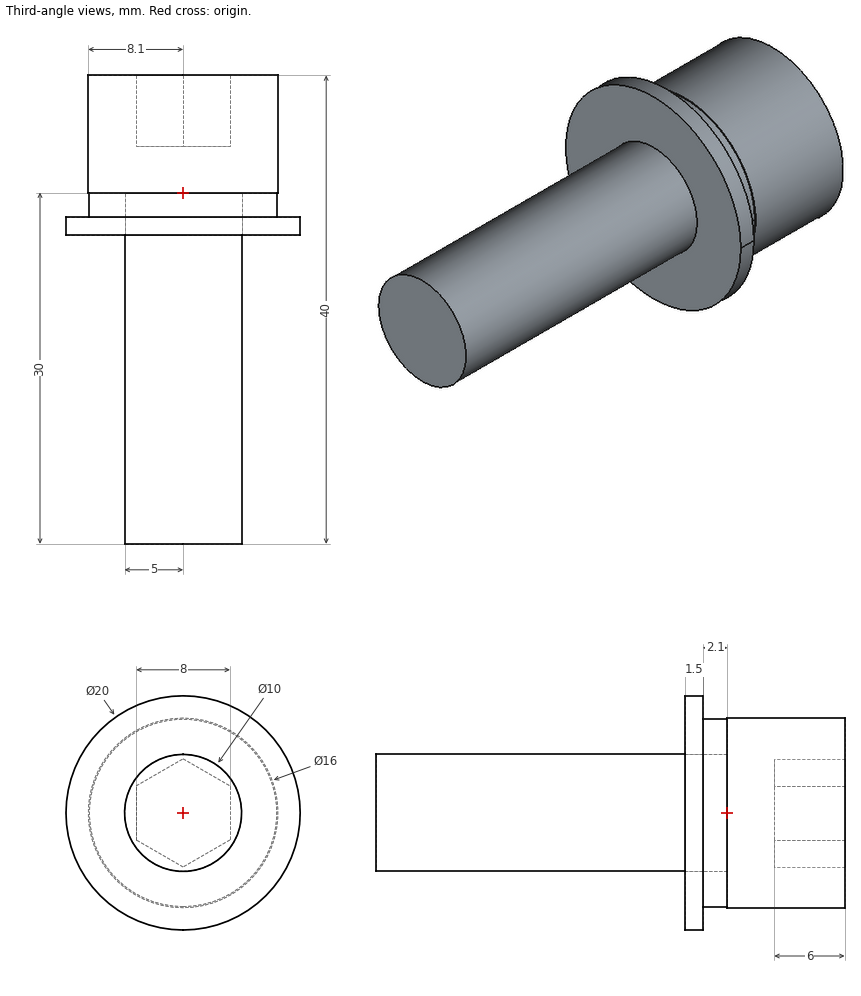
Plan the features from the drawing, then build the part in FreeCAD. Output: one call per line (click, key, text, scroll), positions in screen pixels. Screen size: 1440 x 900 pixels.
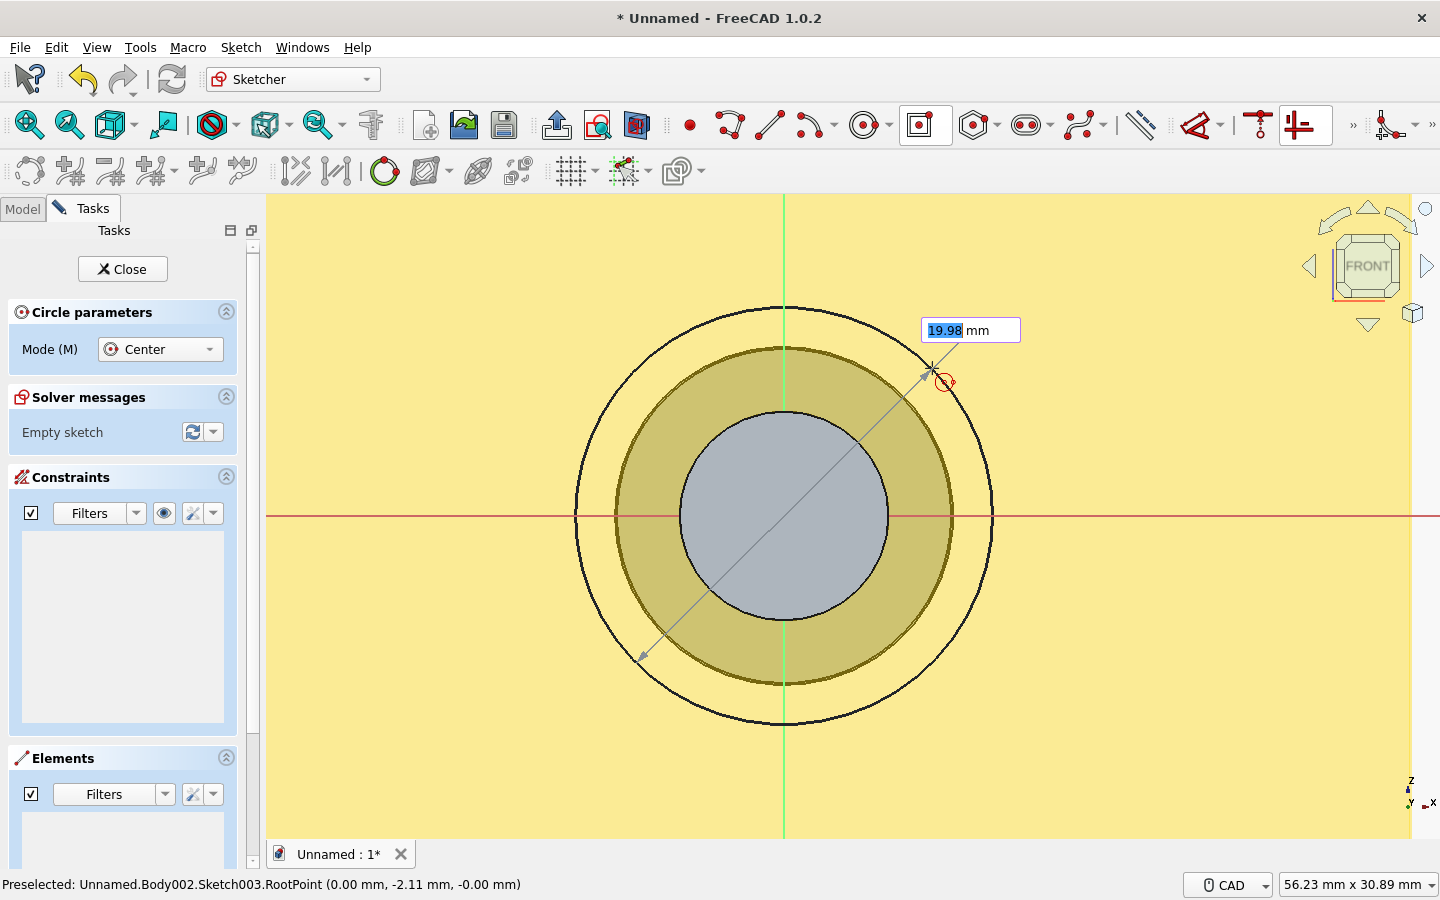
text(20)
key(Return)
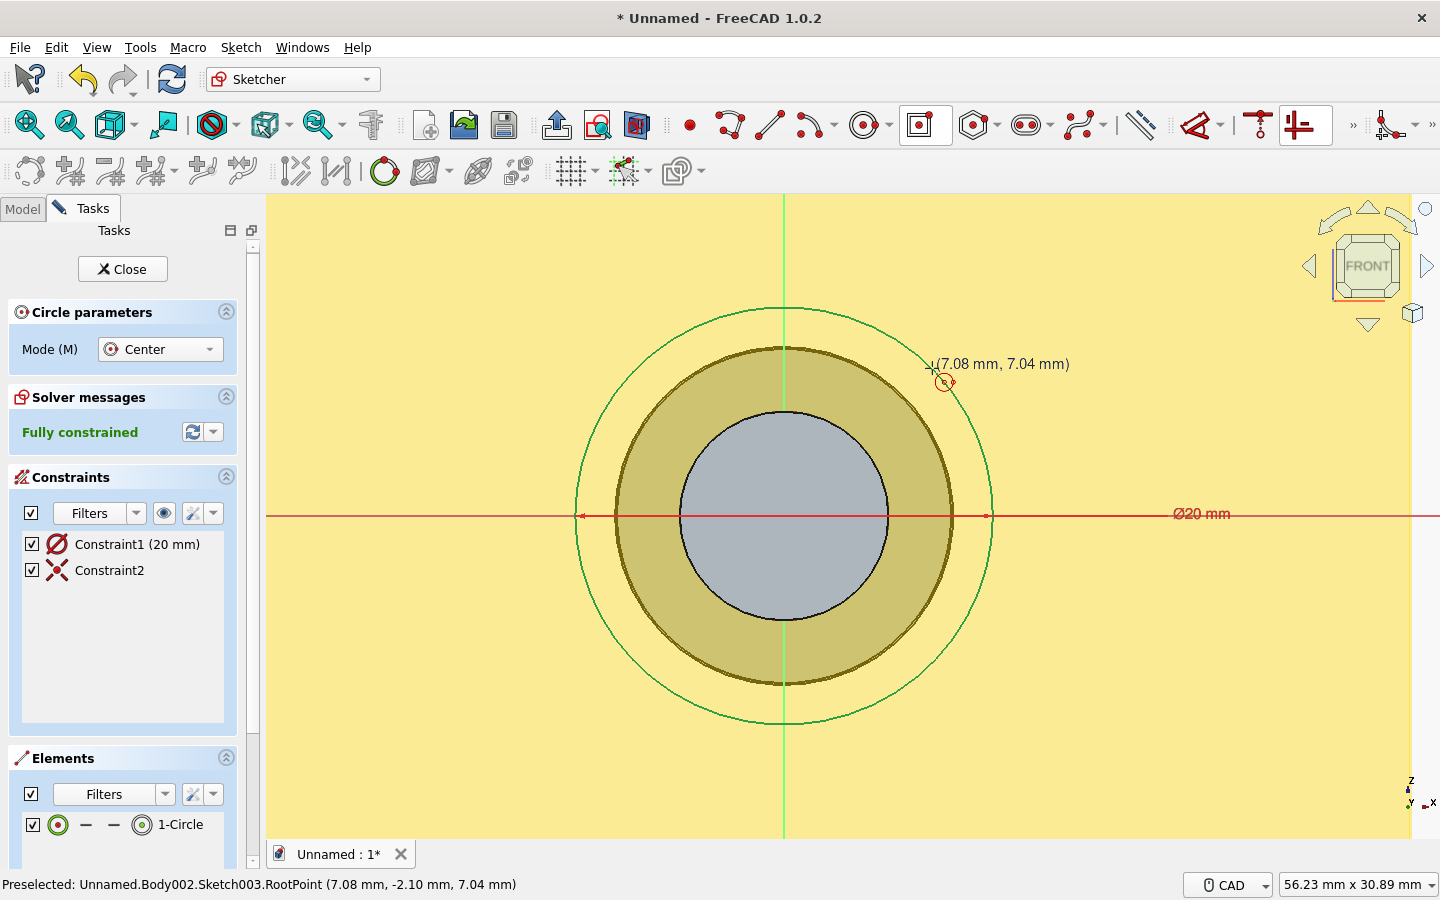
click(784, 516)
move(858, 442)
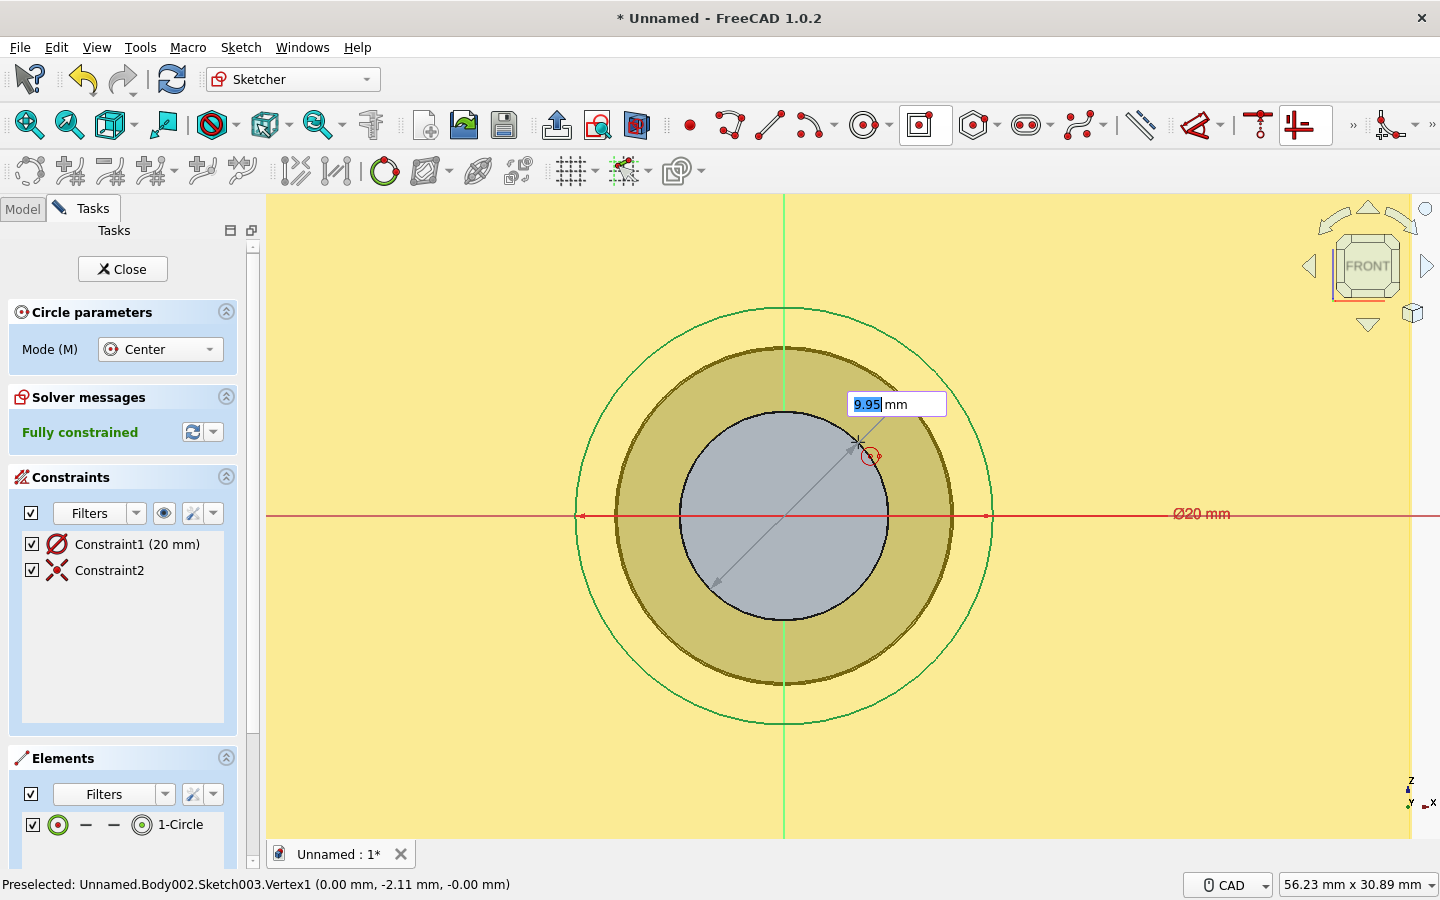
text(10)
key(Return)
key(Escape)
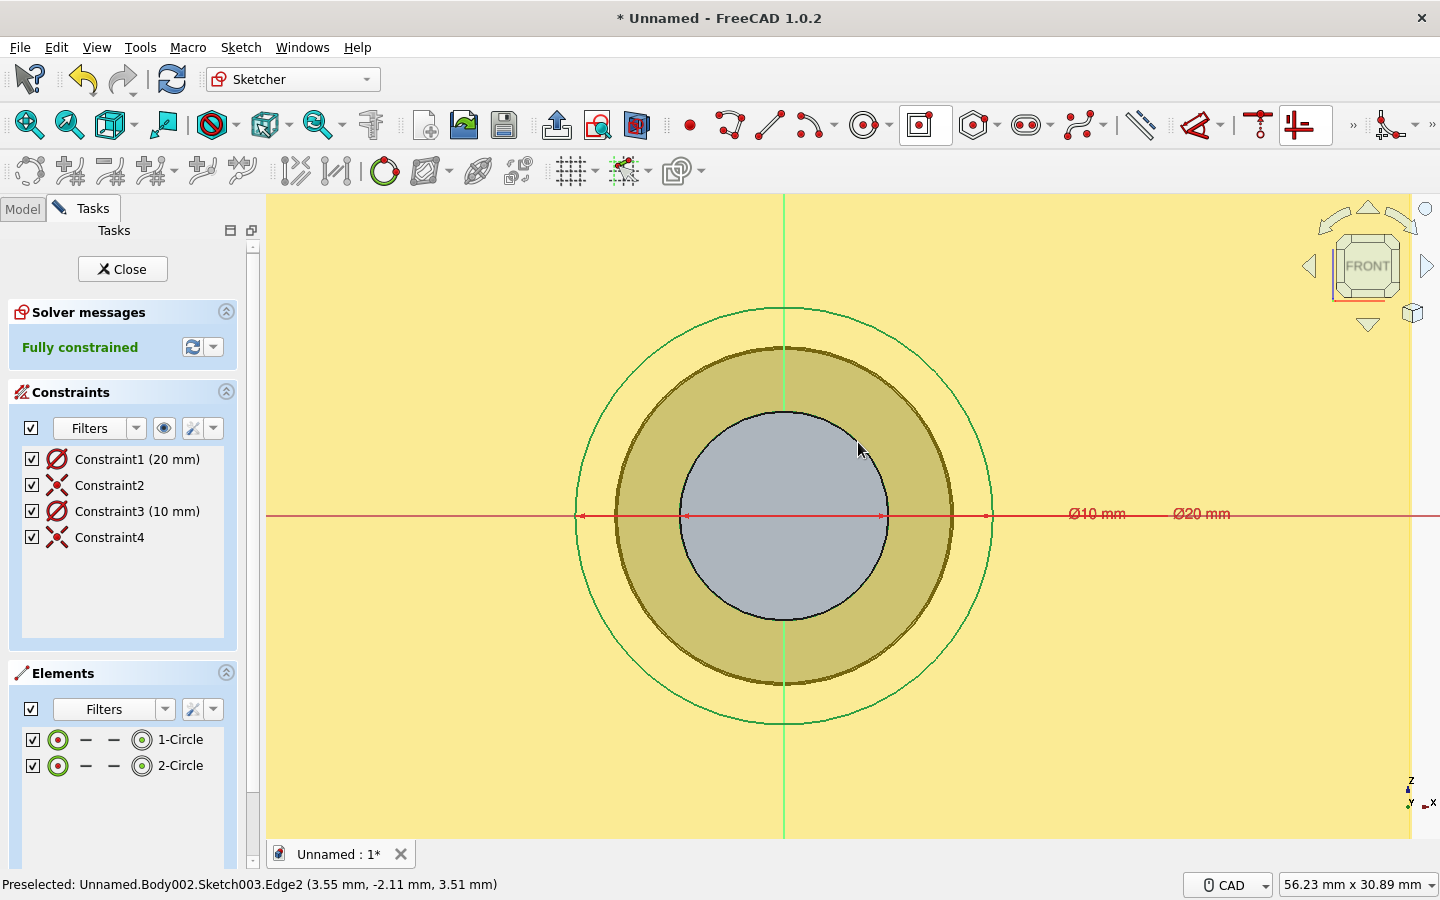
click(123, 269)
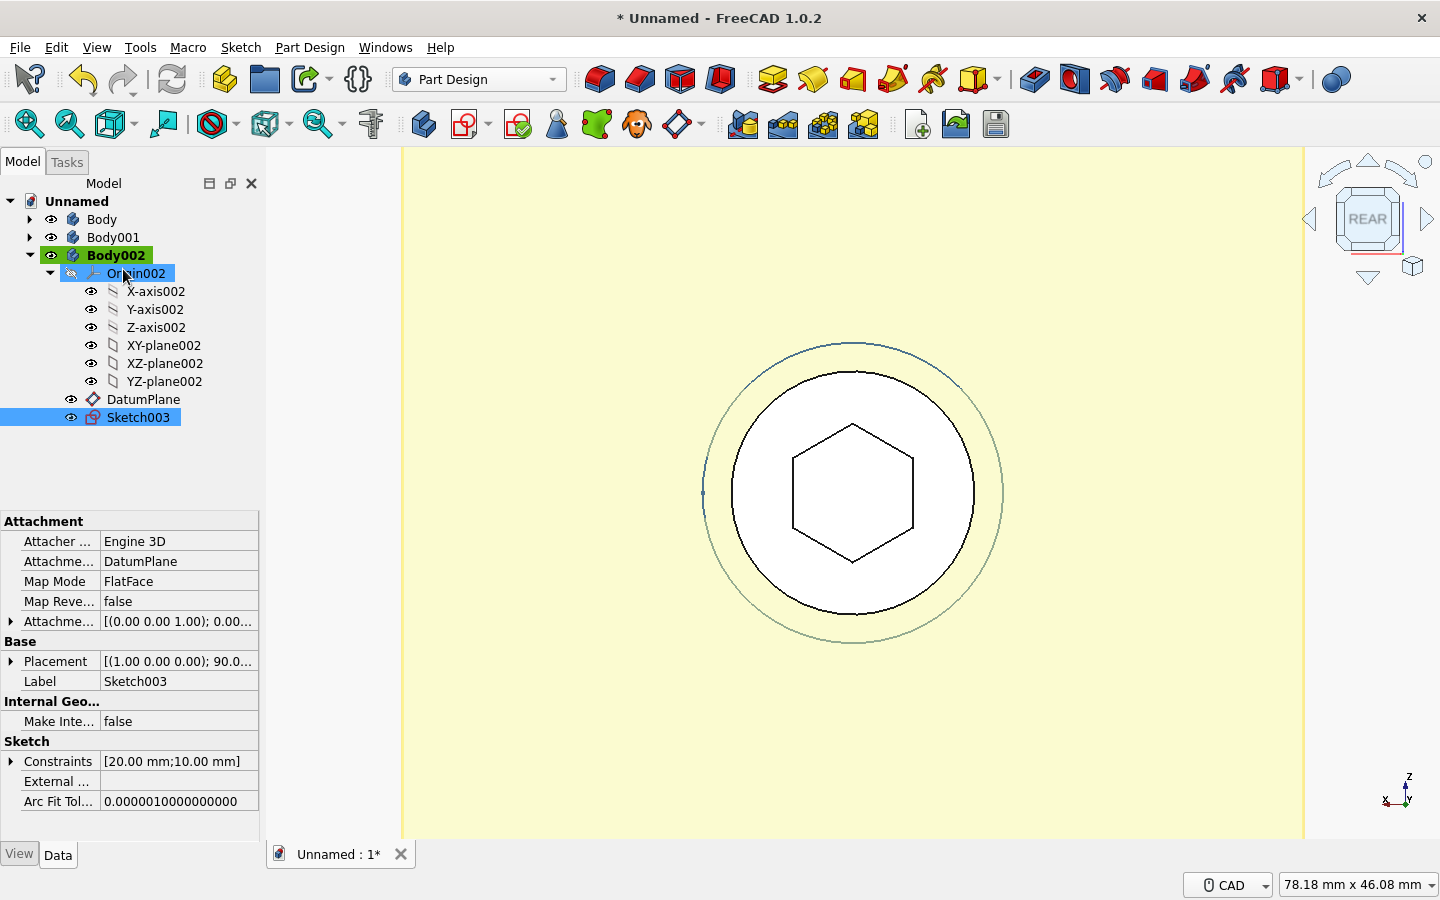
click(774, 80)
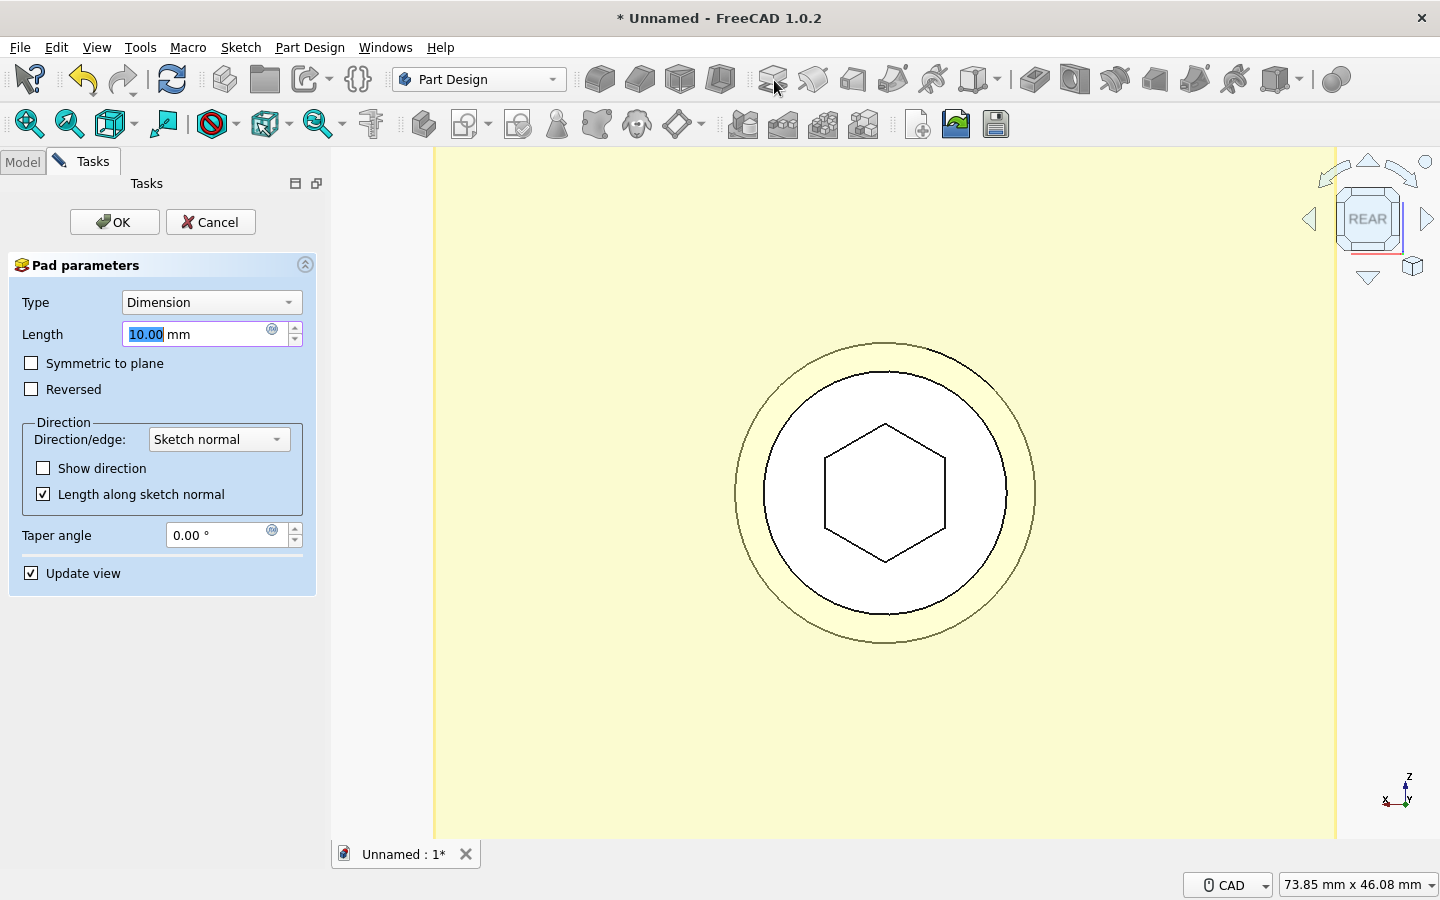
text(1.5)
key(Tab)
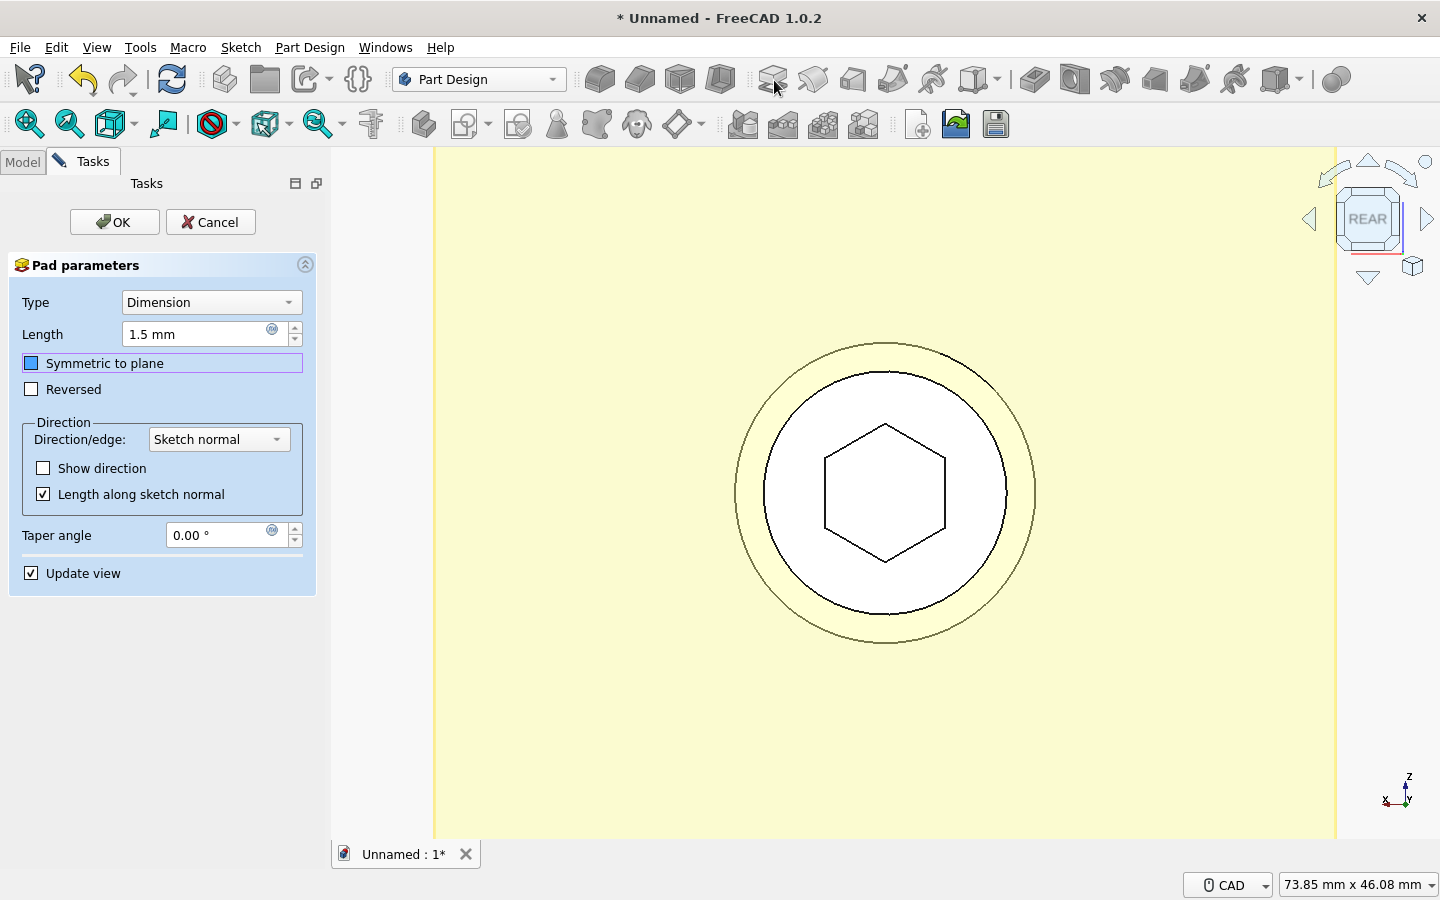
click(115, 222)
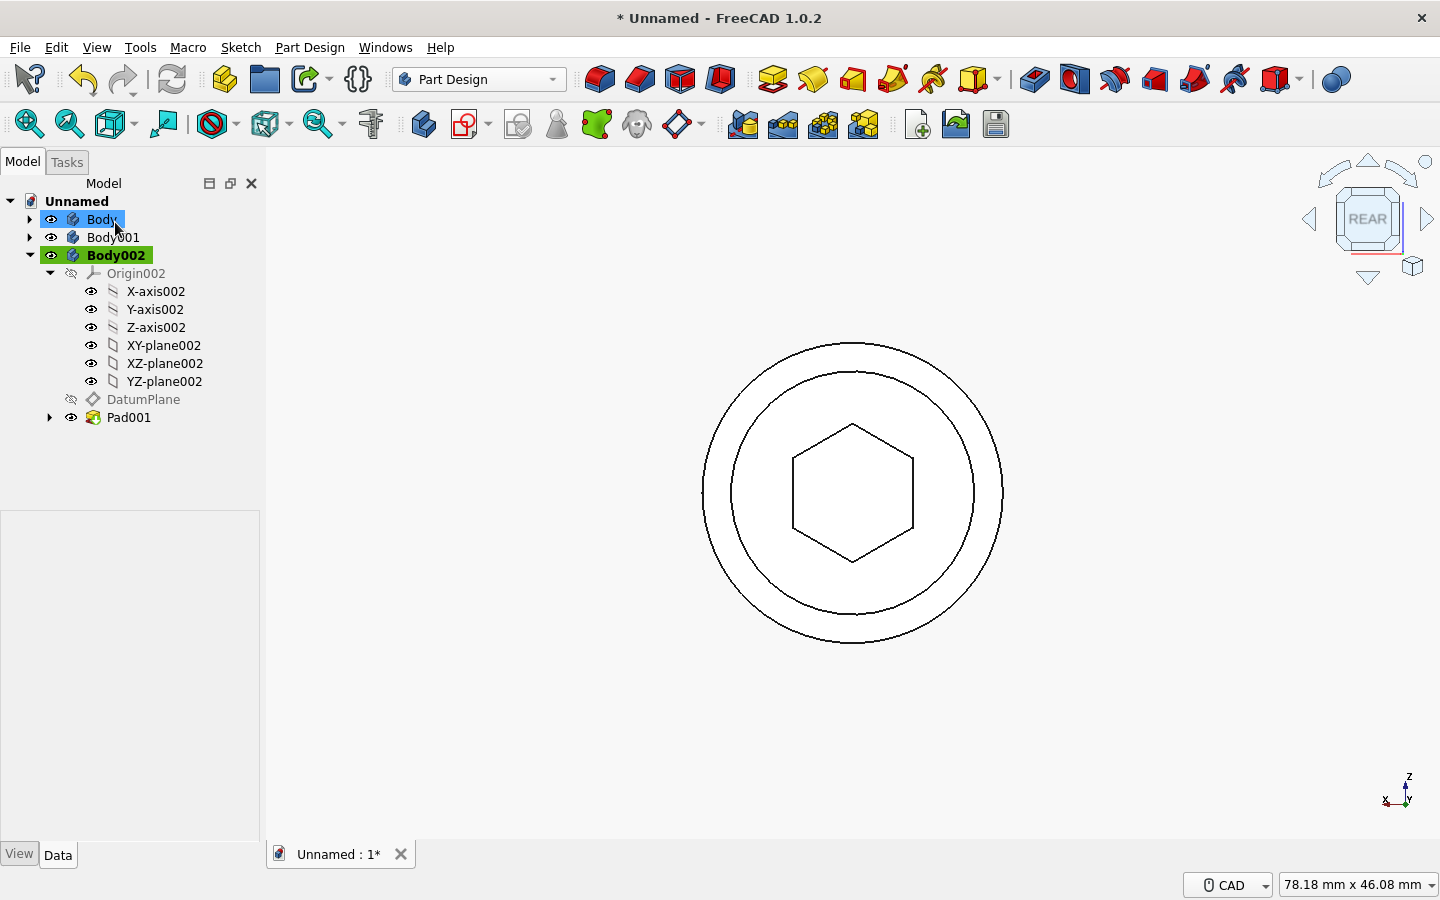
key(0)